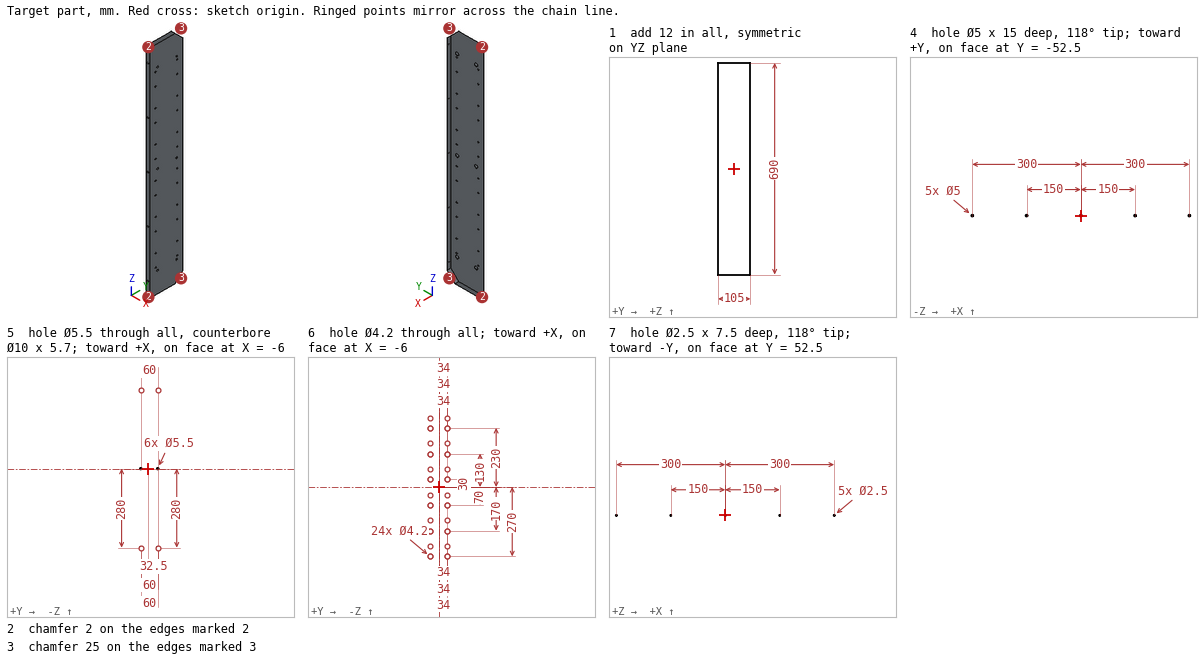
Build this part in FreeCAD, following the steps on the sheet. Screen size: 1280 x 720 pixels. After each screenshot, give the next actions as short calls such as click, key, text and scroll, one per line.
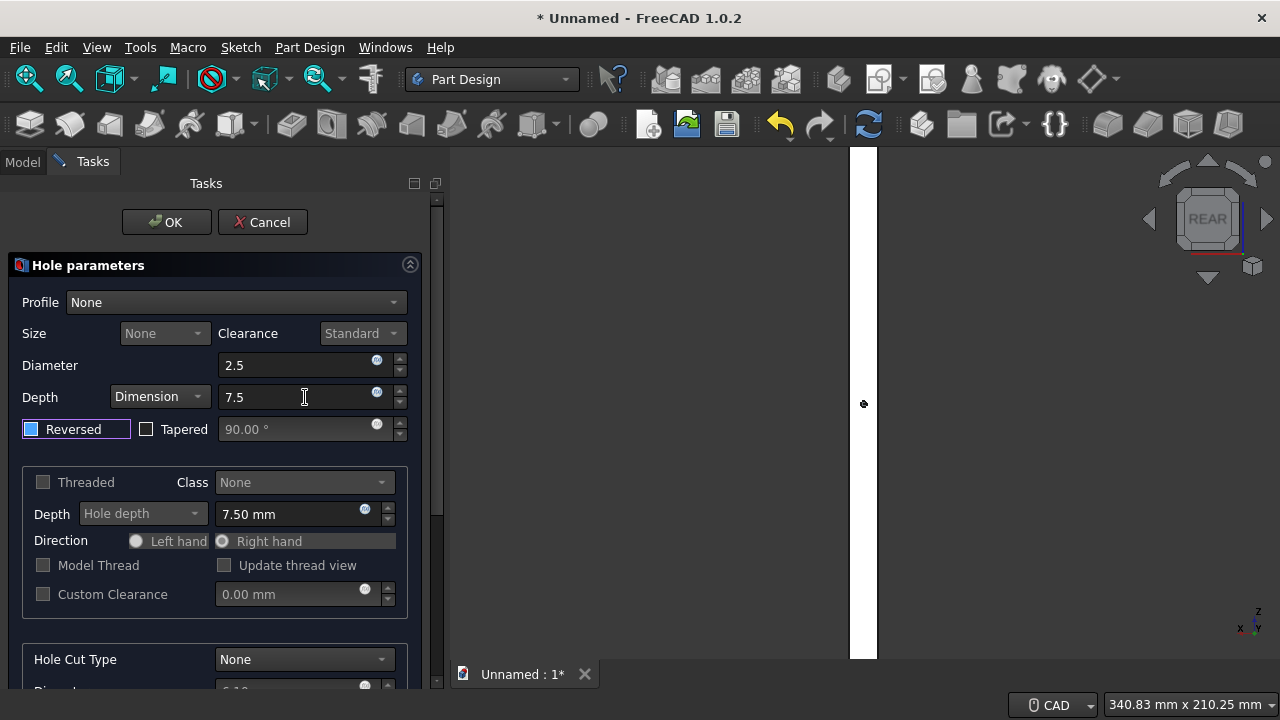
click(167, 222)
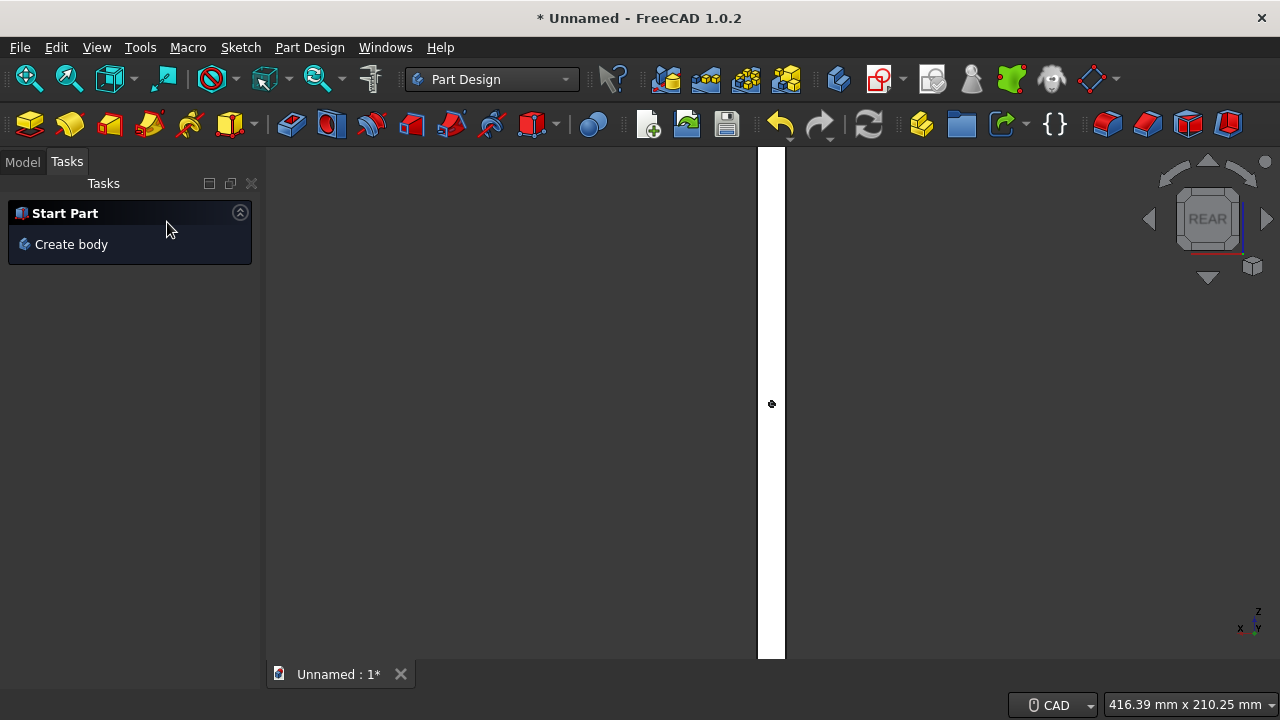
key(0)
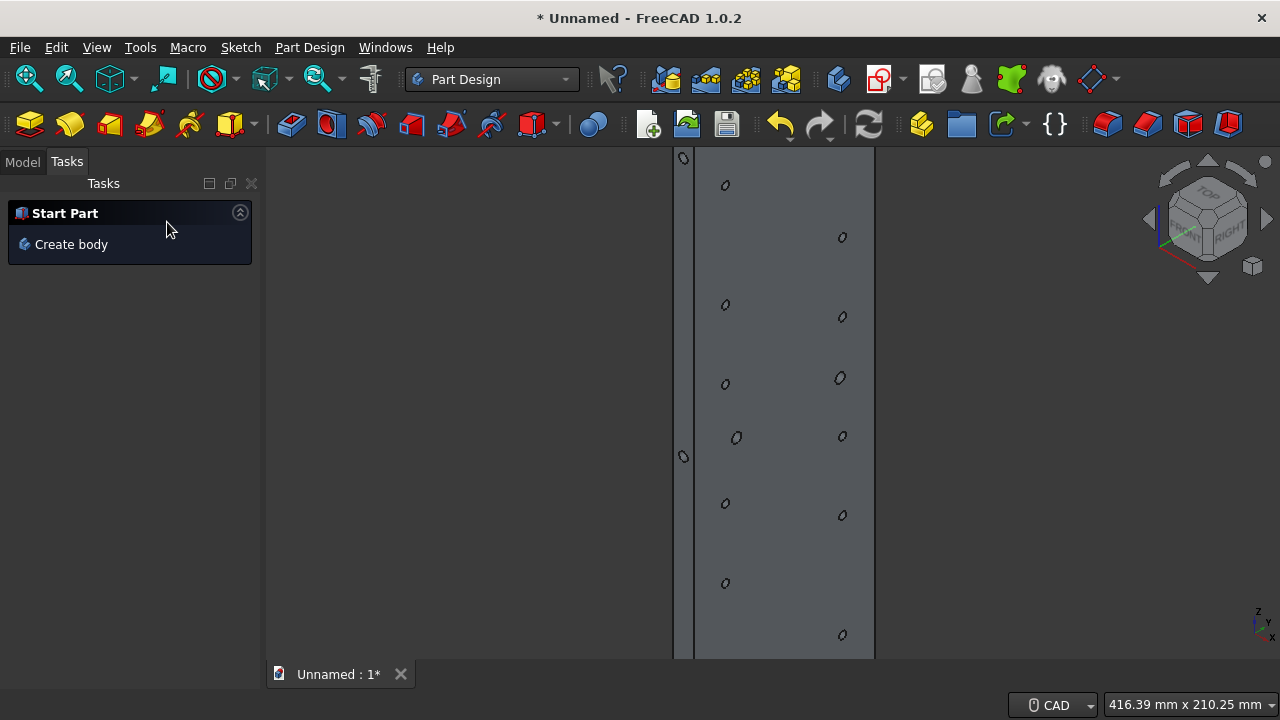
click(30, 80)